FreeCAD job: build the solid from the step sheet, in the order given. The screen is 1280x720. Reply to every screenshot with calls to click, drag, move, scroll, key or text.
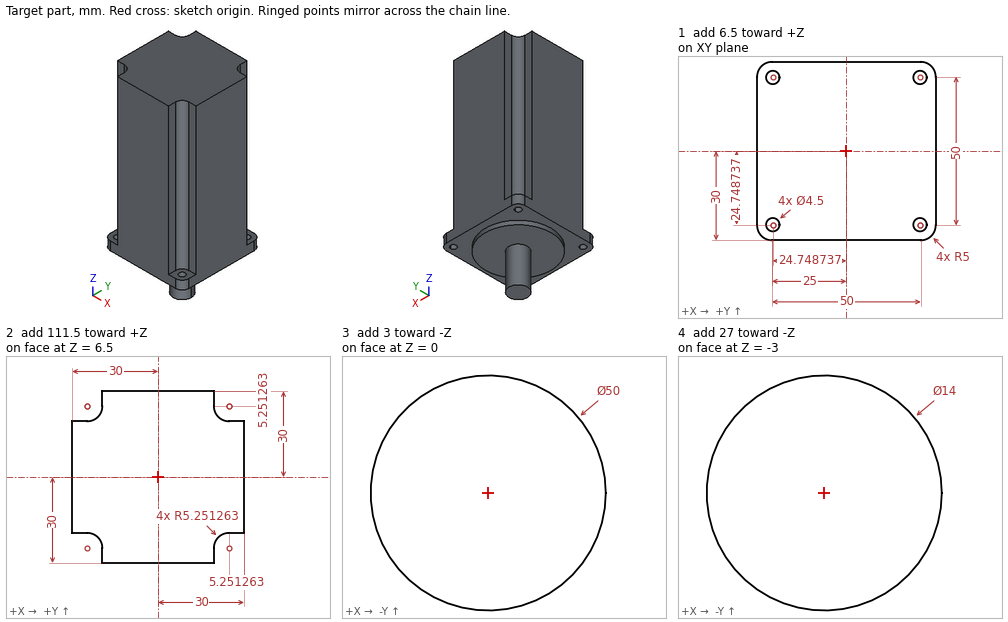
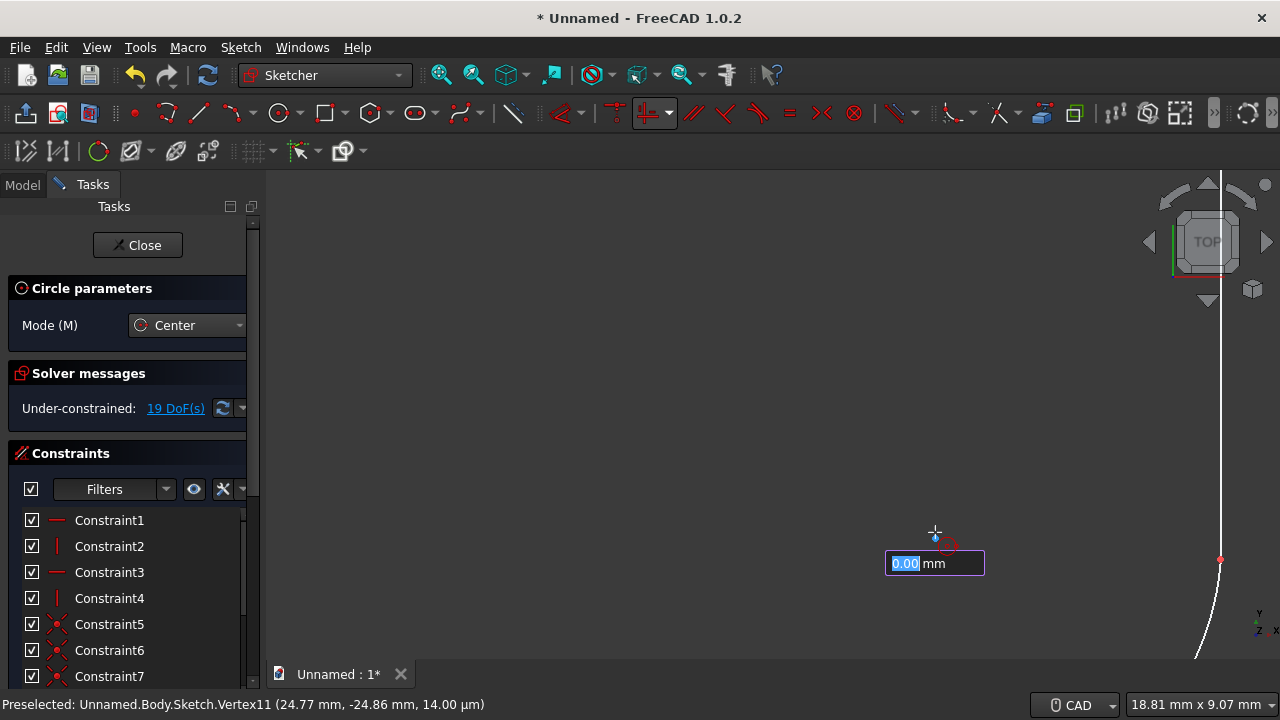
scroll(815, 536, down, 12)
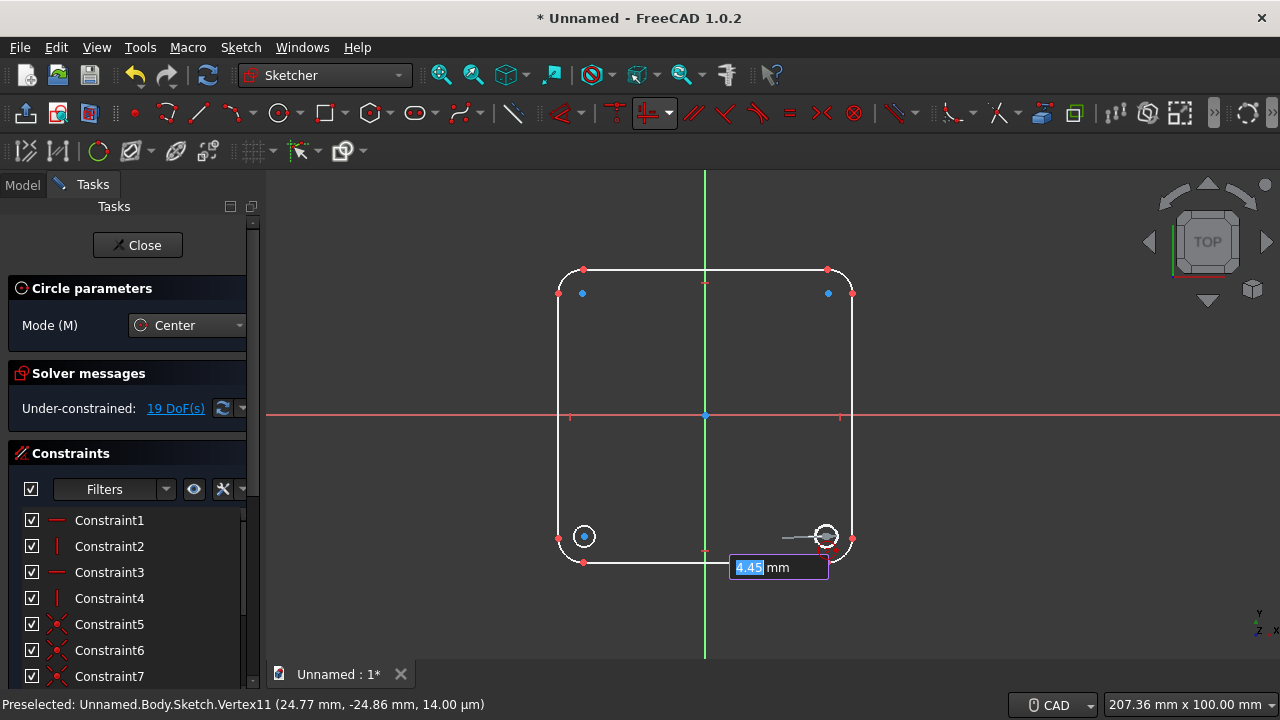
scroll(834, 529, up, 2)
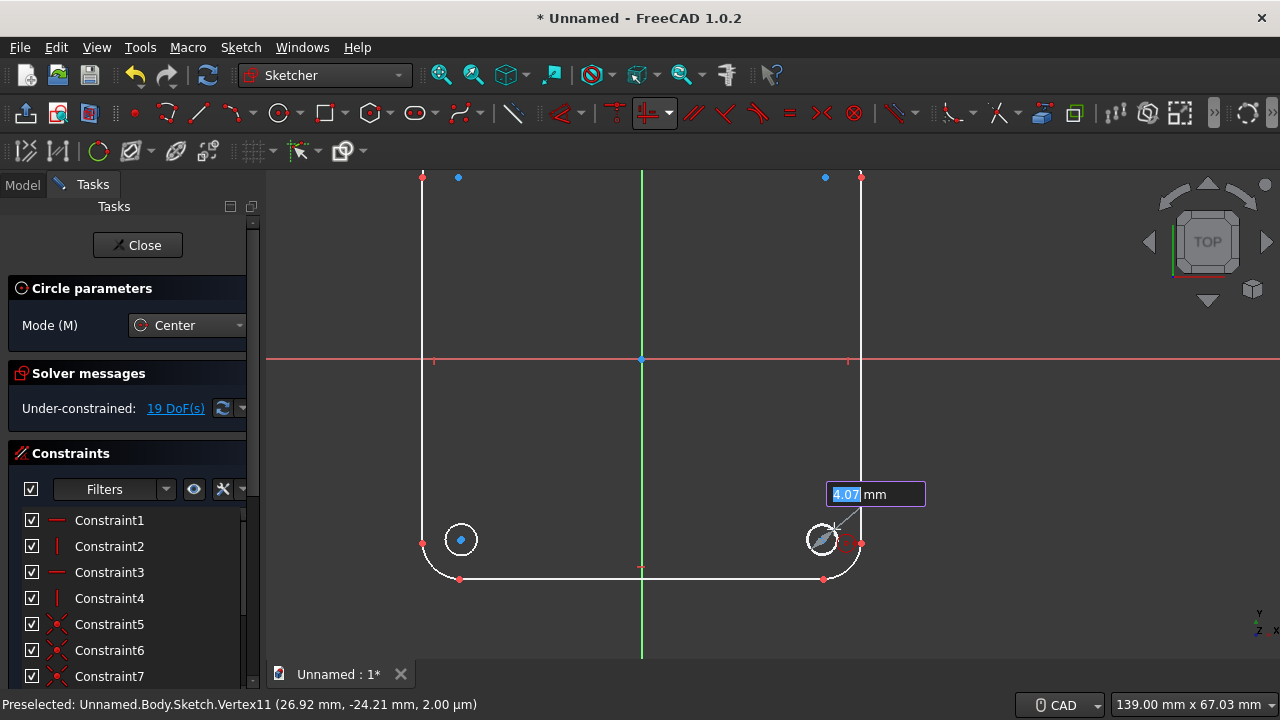
click(834, 528)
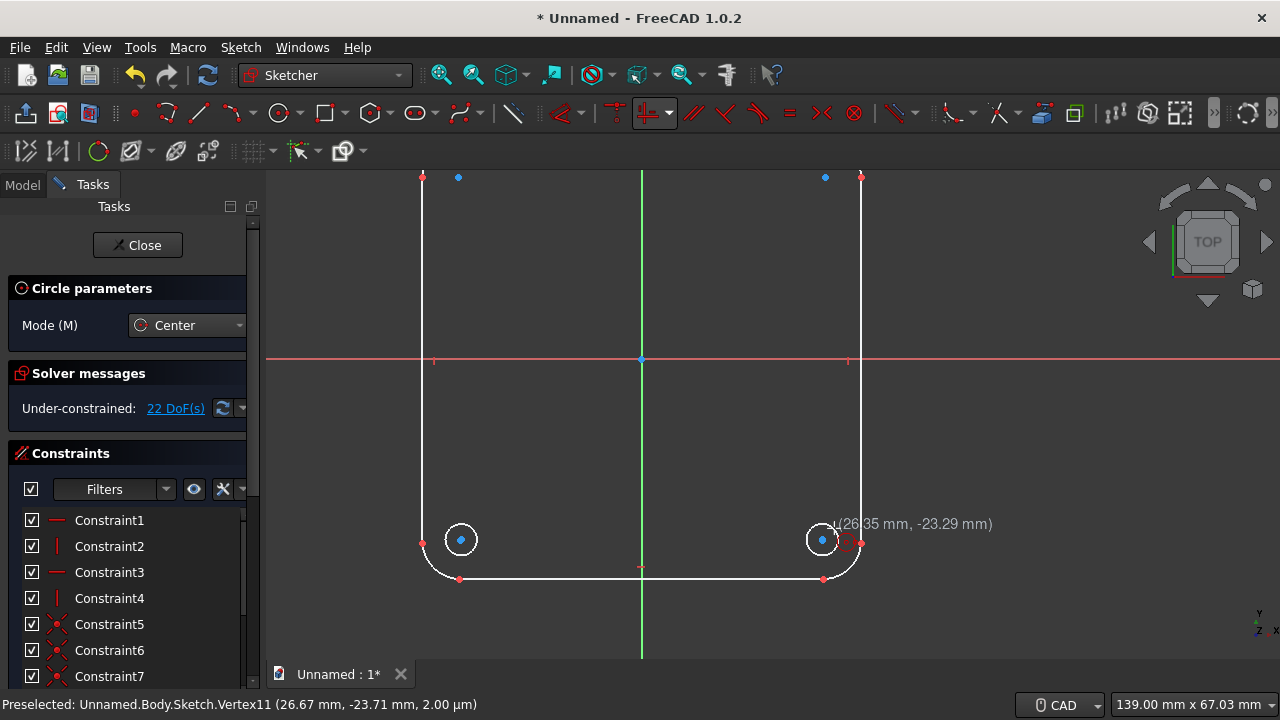
scroll(832, 527, down, 2)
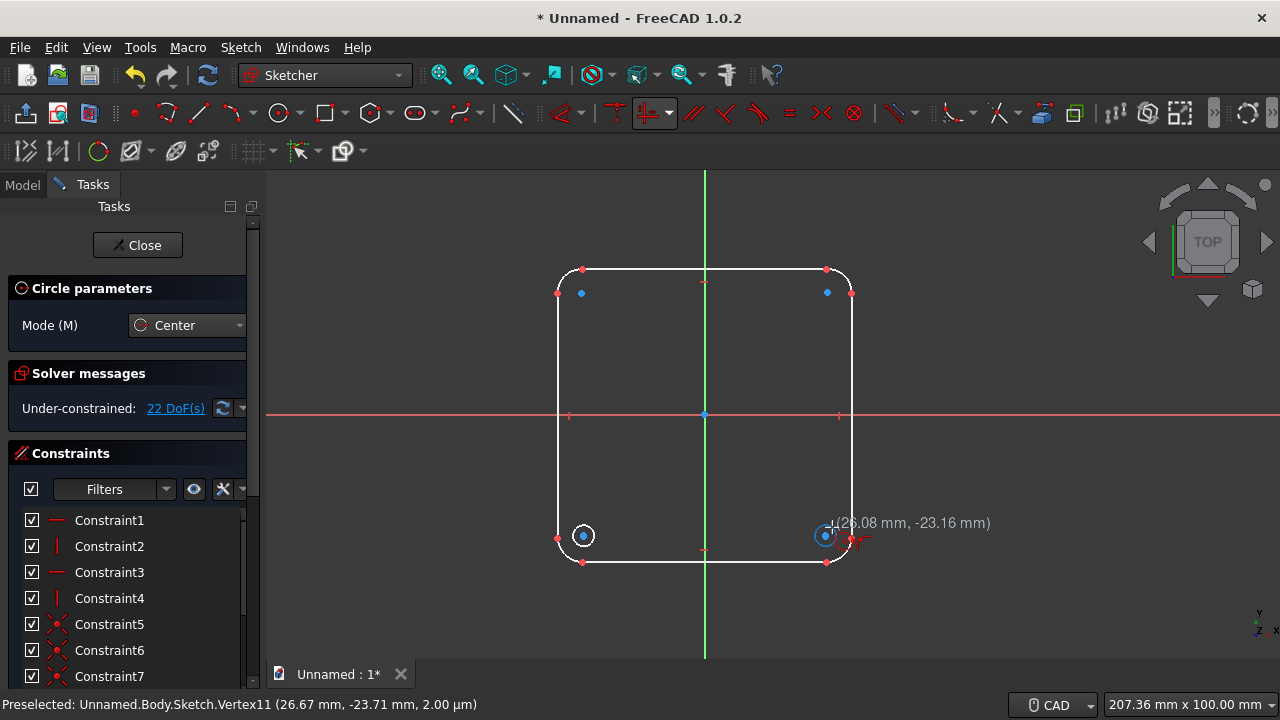
scroll(584, 294, up, 12)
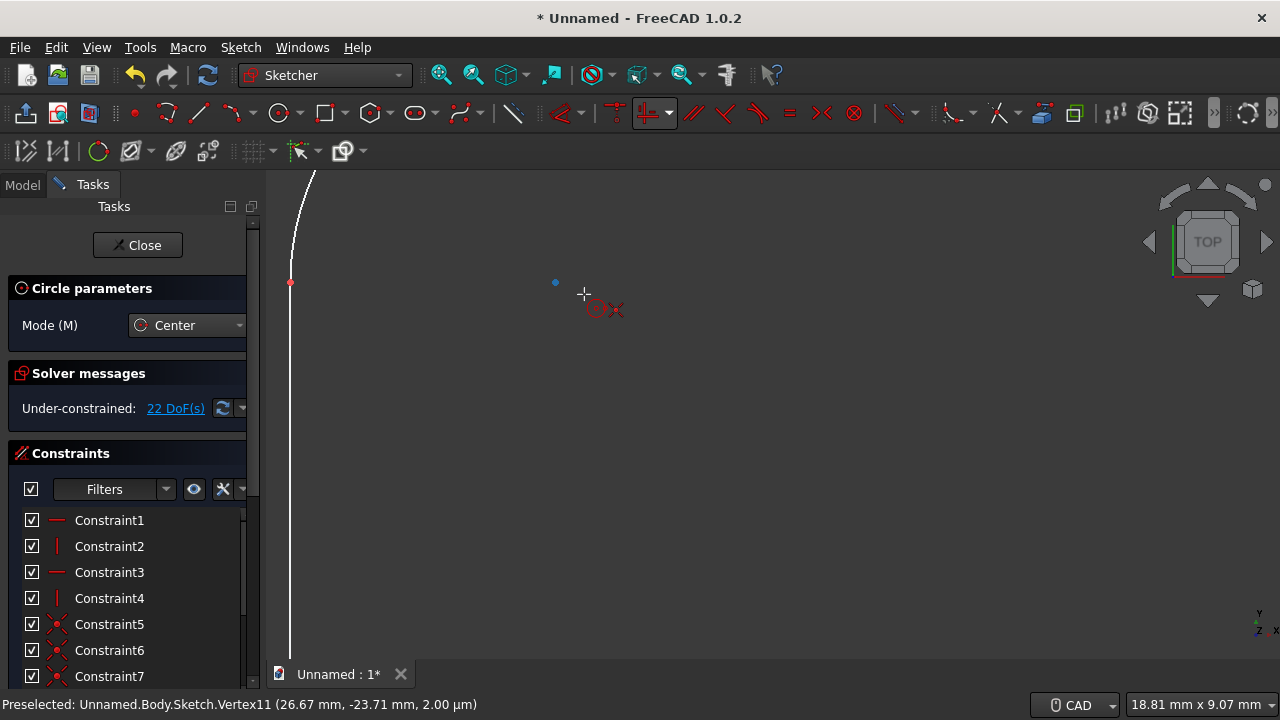
click(577, 288)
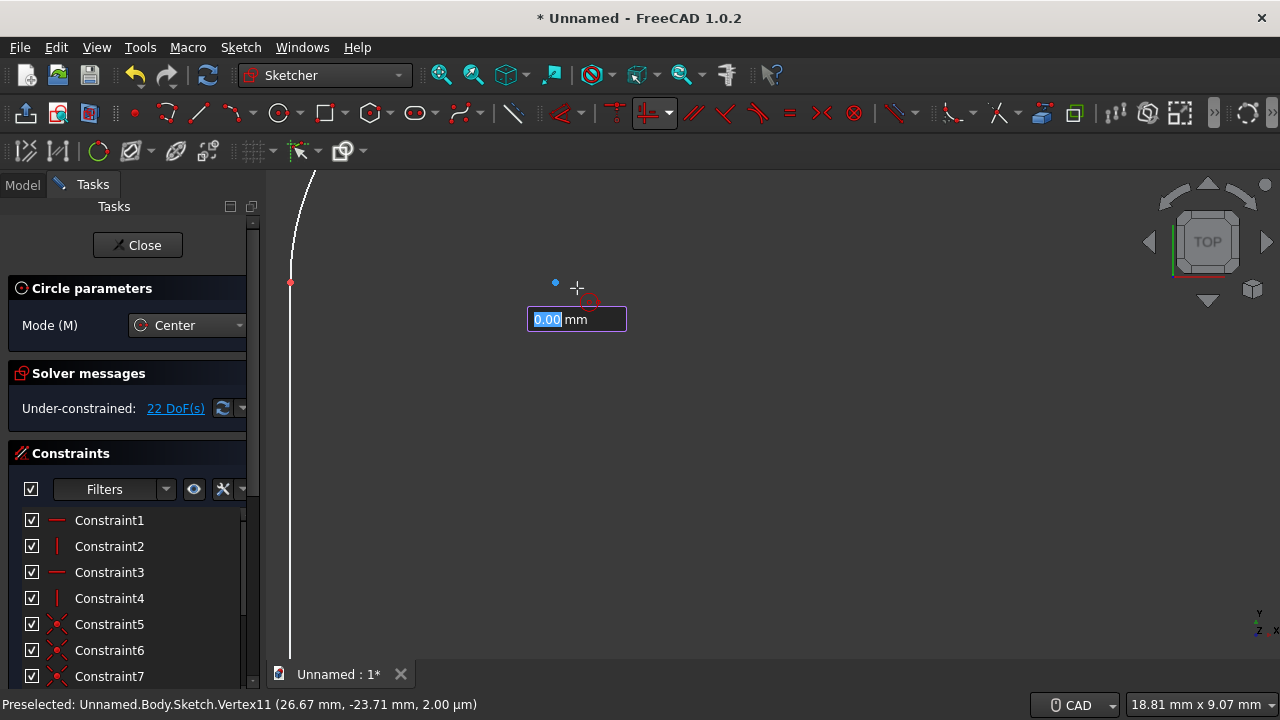
scroll(584, 294, down, 12)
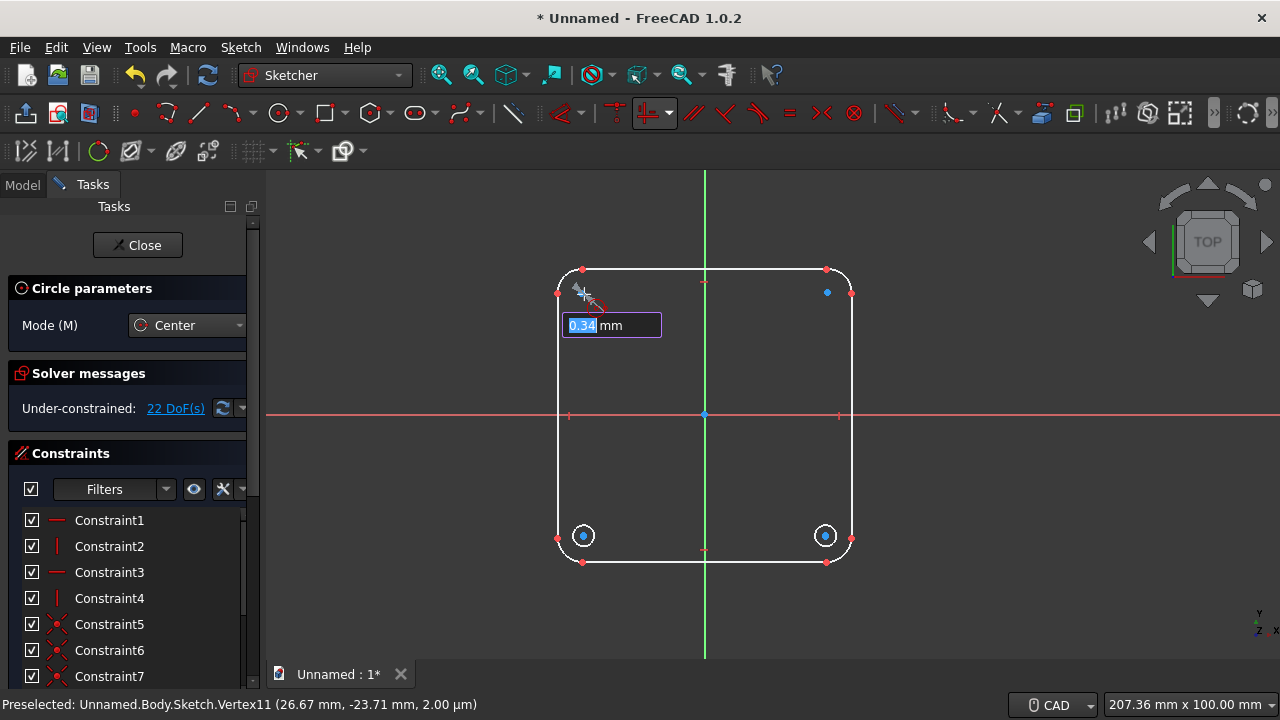
scroll(591, 286, up, 2)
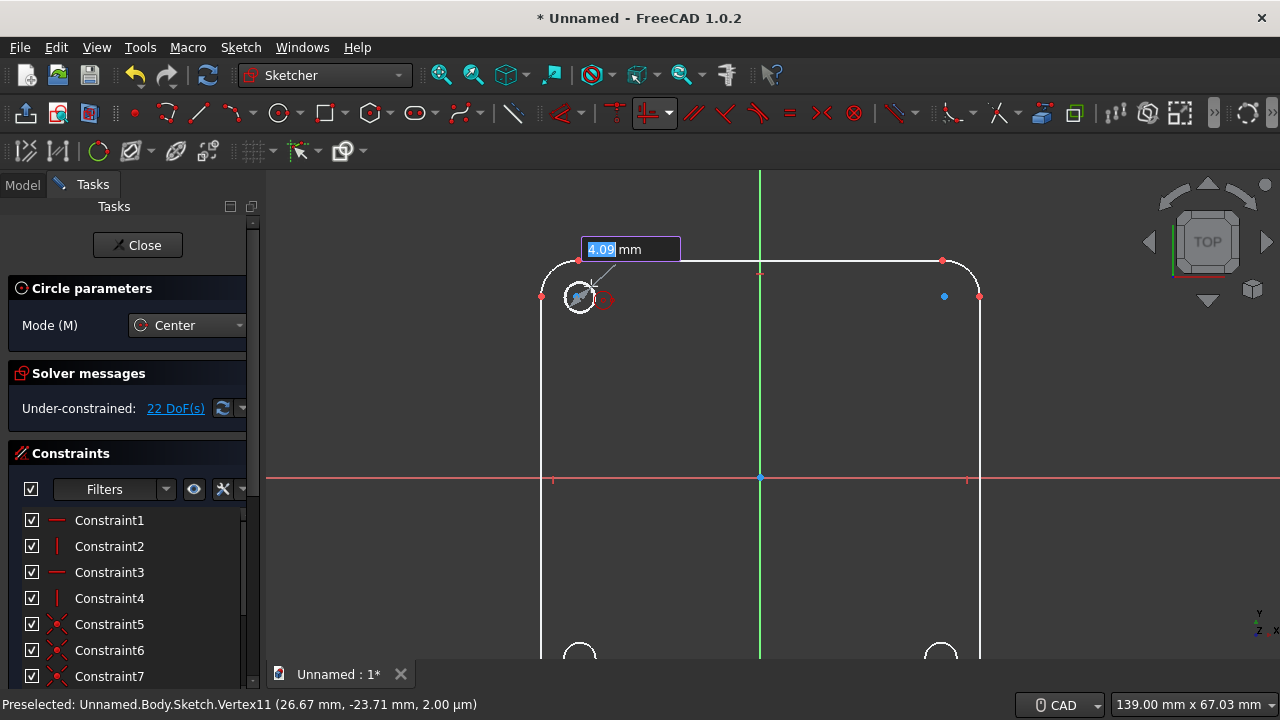
click(591, 286)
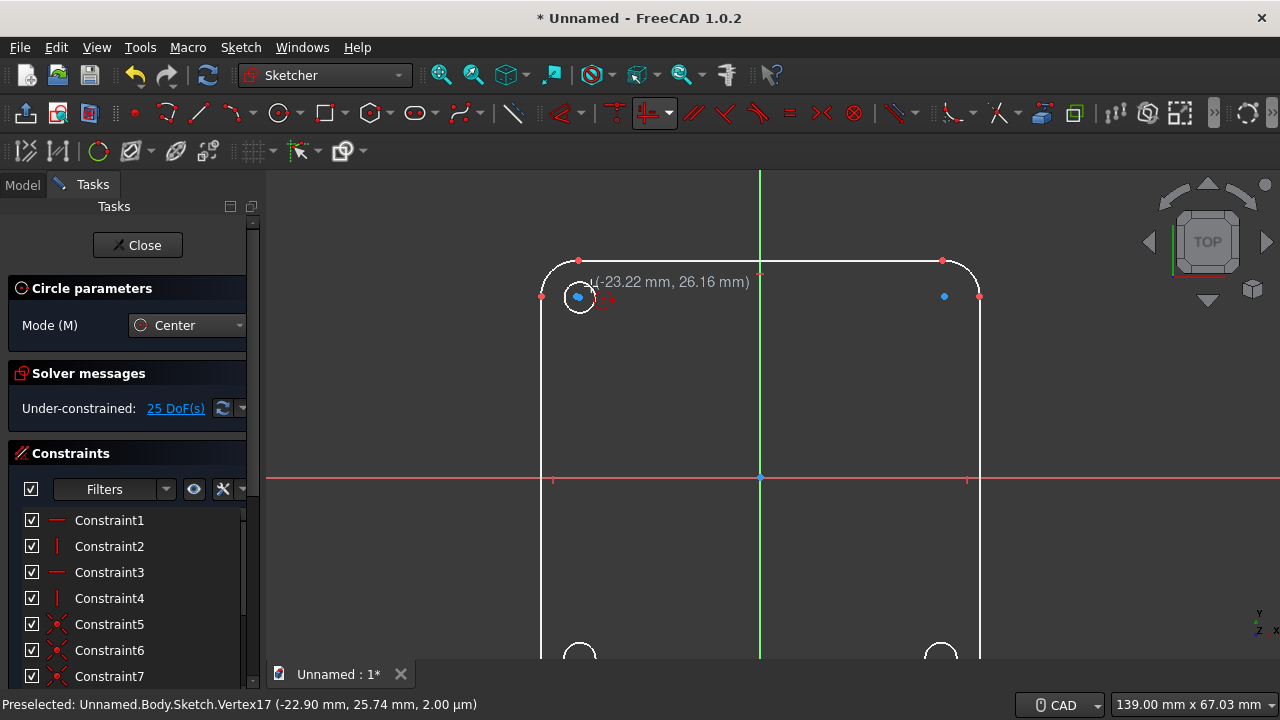
scroll(941, 297, up, 10)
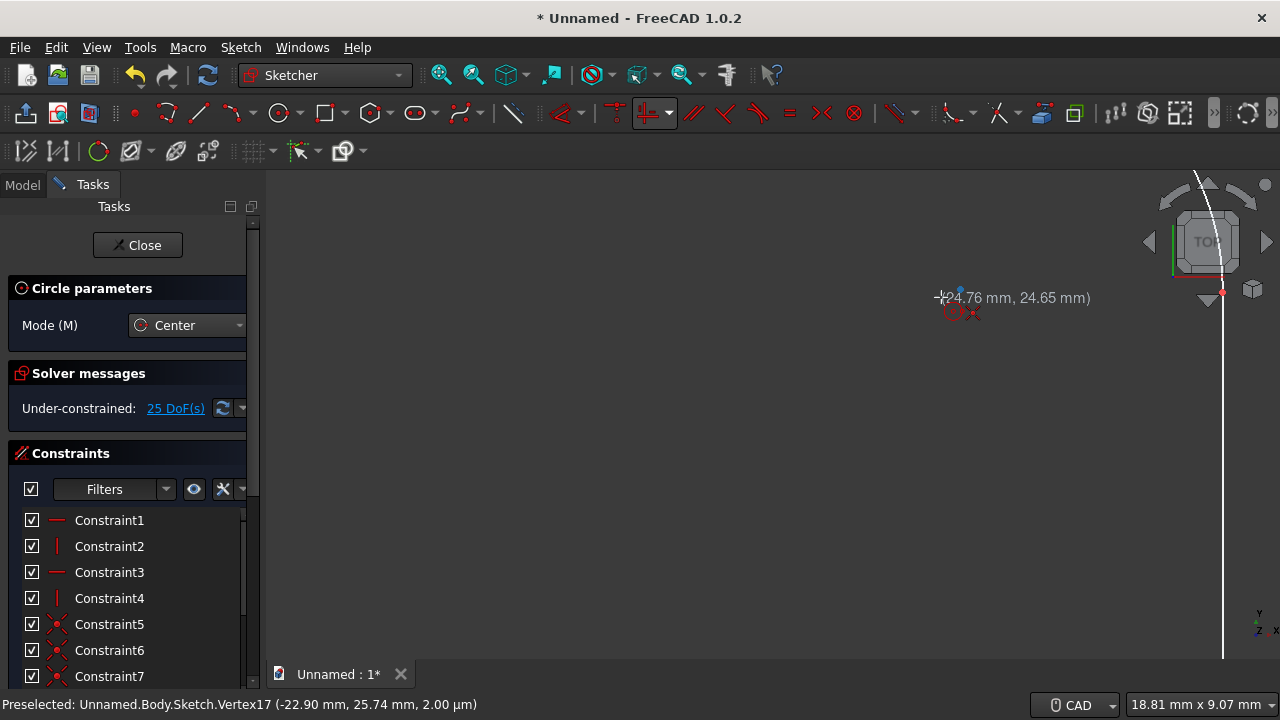
click(936, 298)